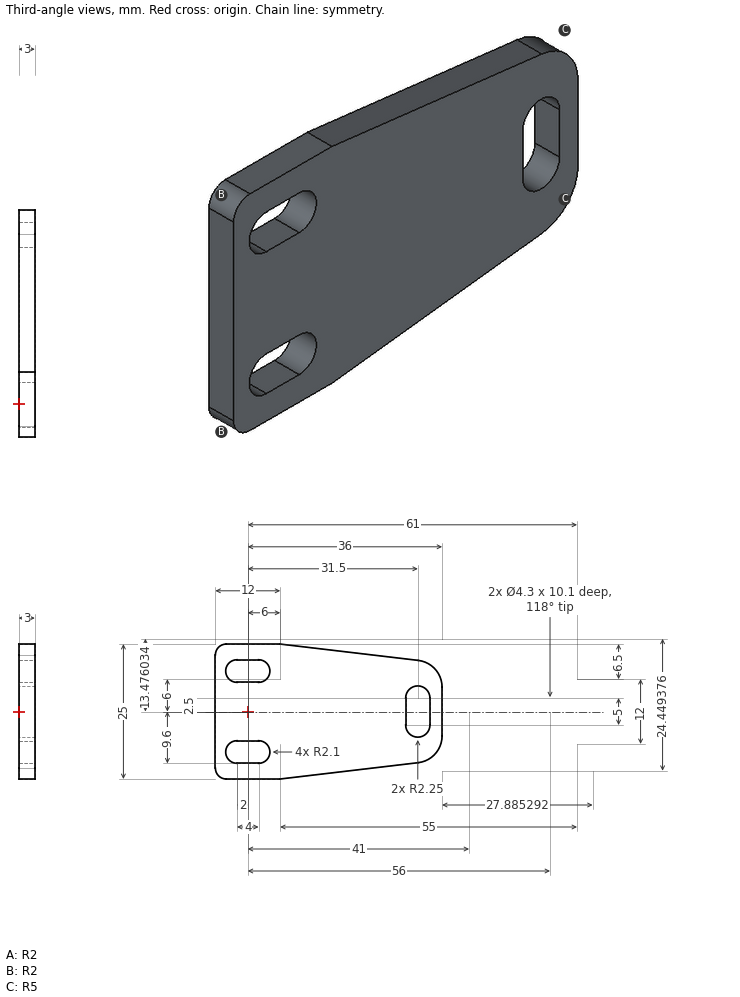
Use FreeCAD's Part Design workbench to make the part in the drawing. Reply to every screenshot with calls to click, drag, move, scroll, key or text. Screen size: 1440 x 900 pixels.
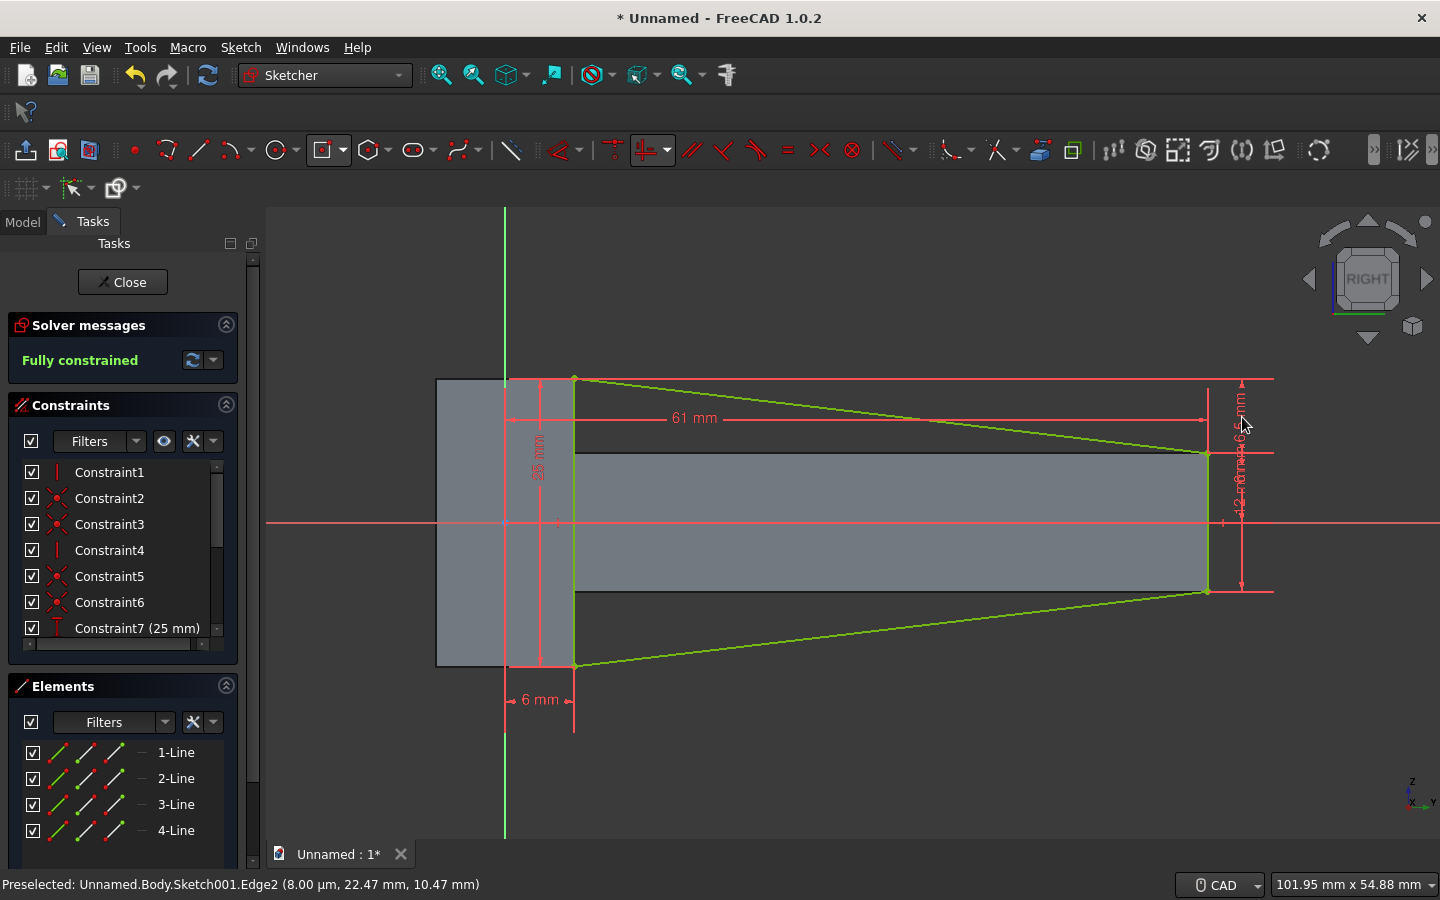
click(123, 282)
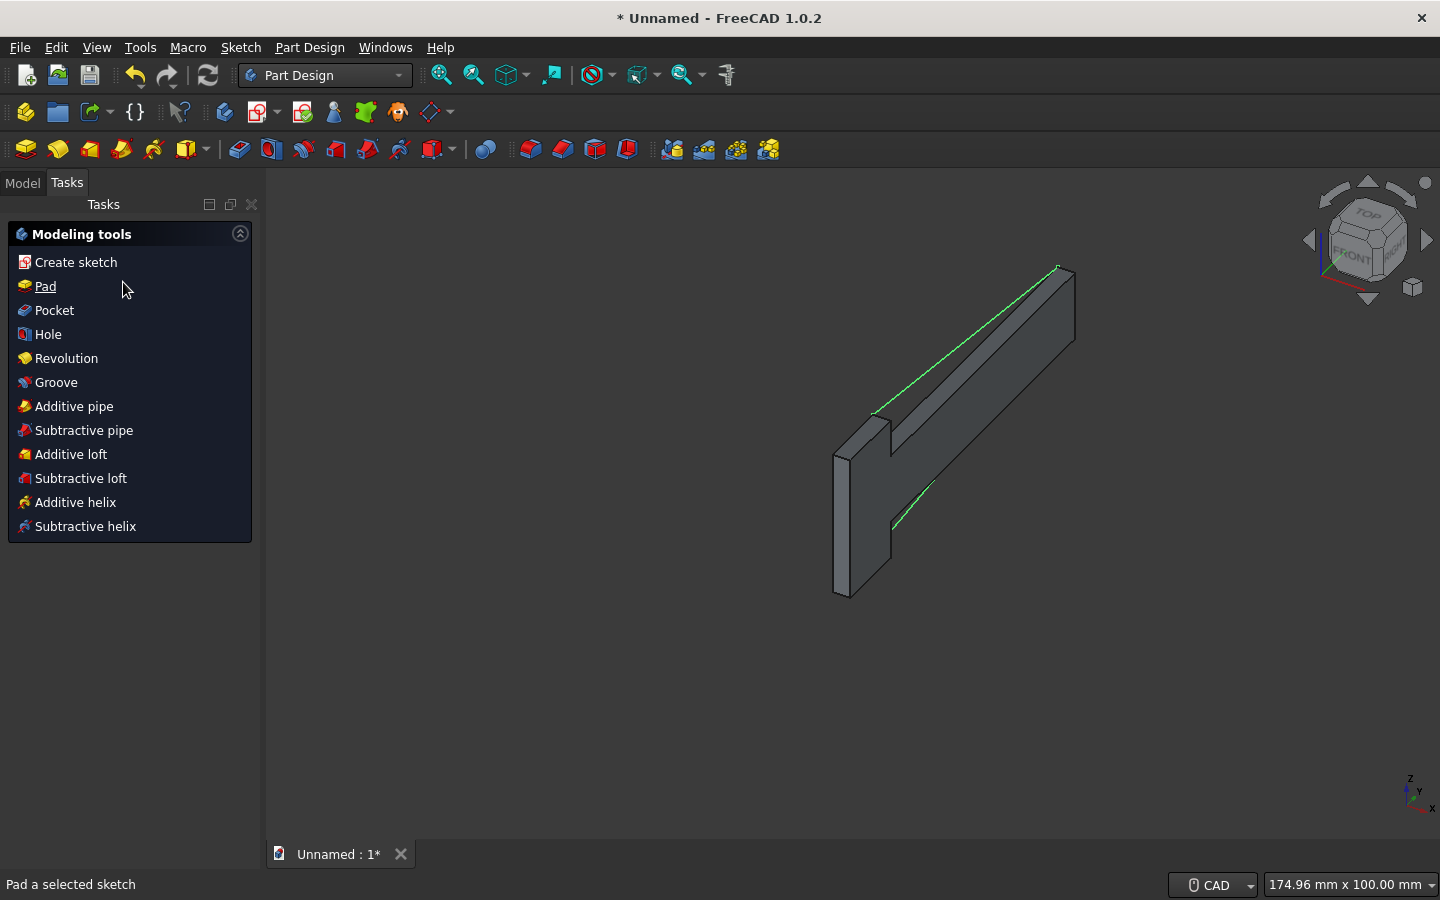
click(26, 150)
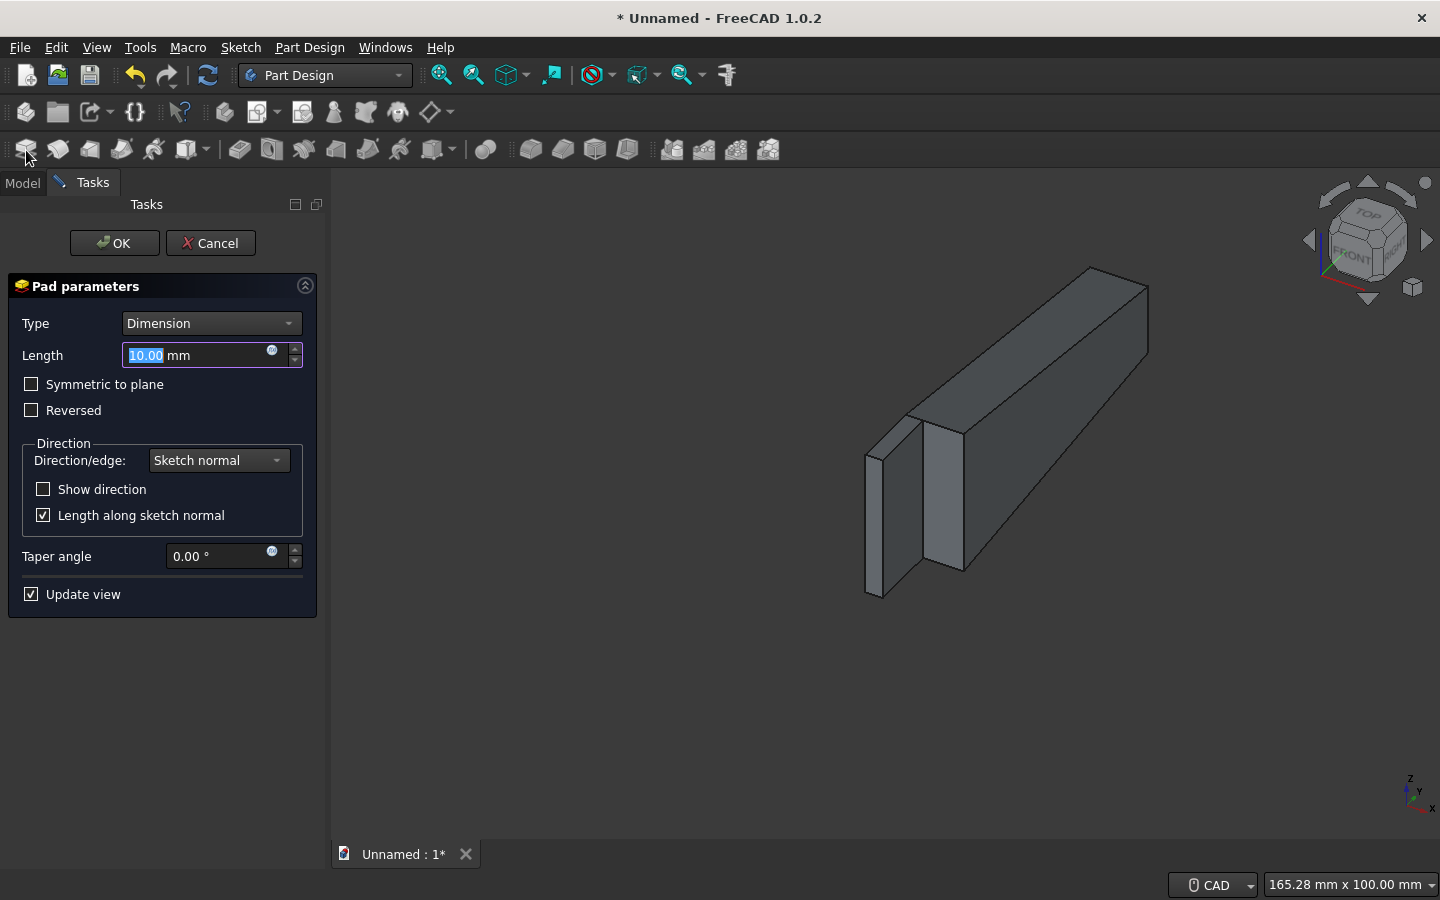
text(3)
key(Tab)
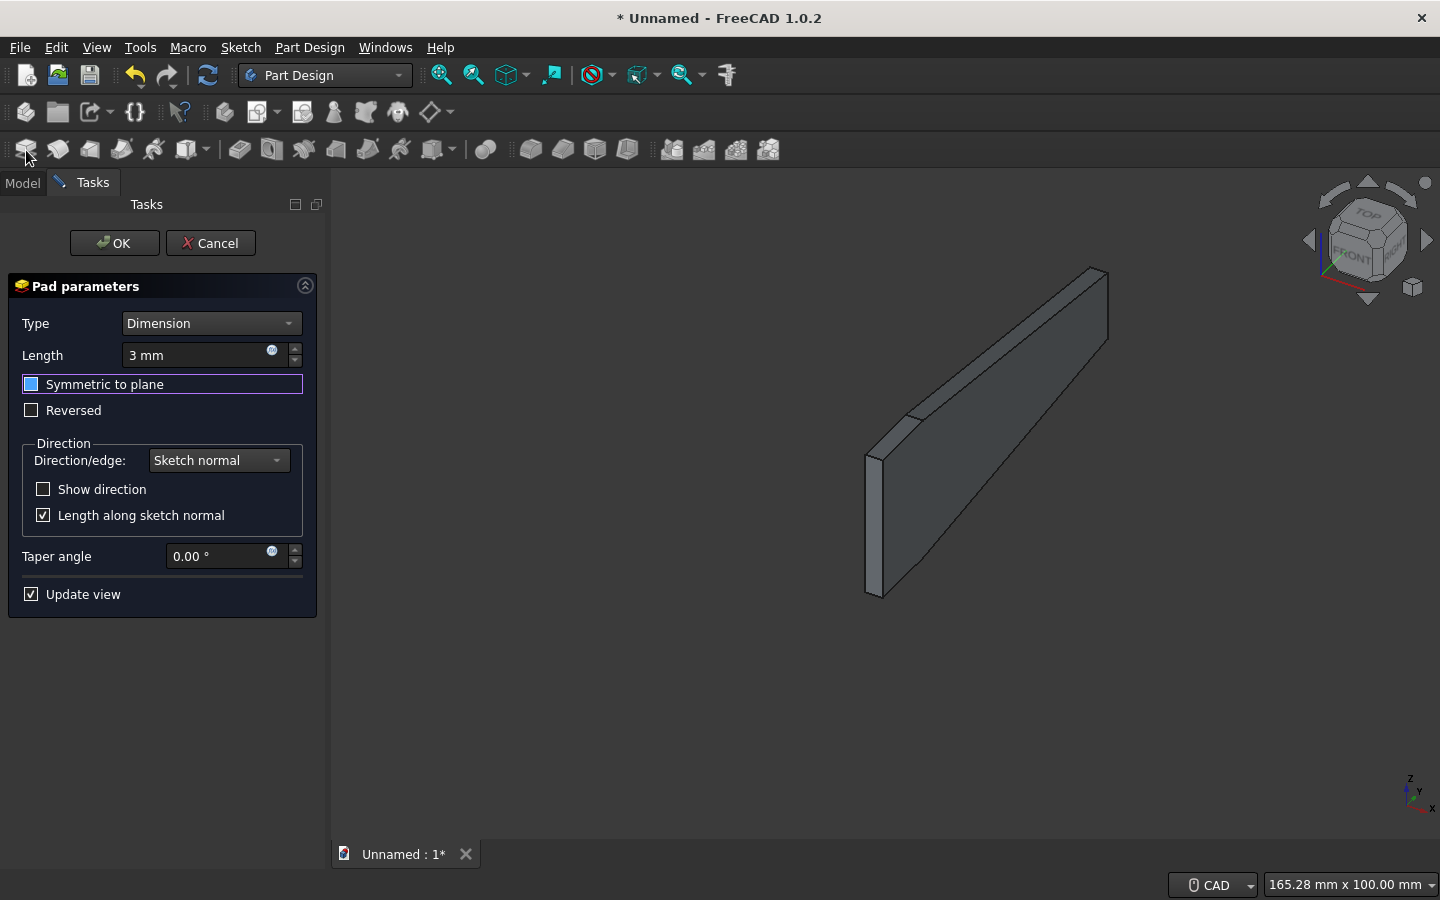
click(115, 243)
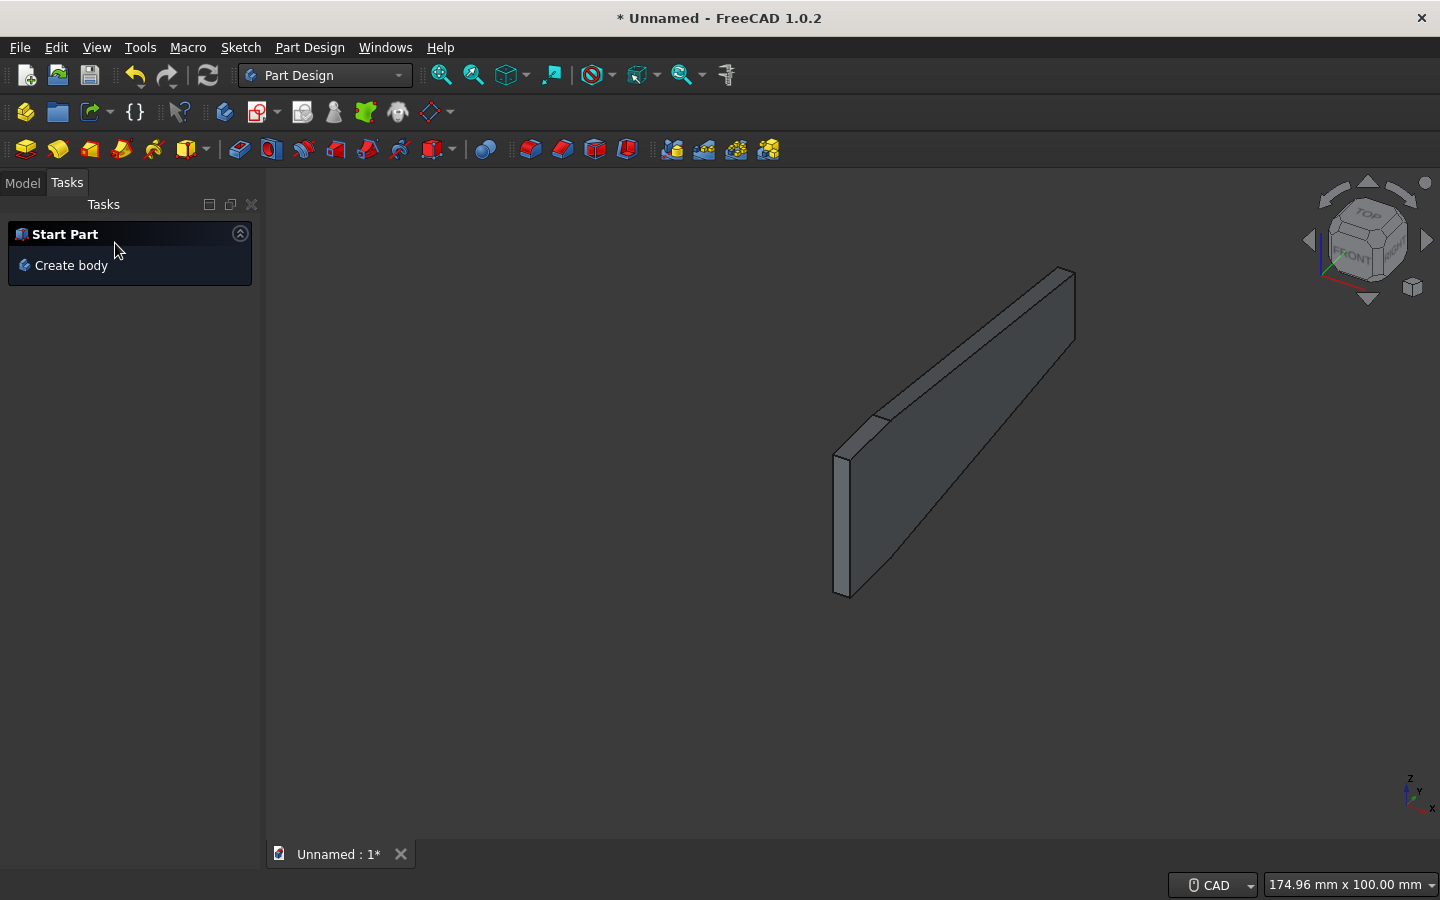
scroll(1066, 269, up, 4)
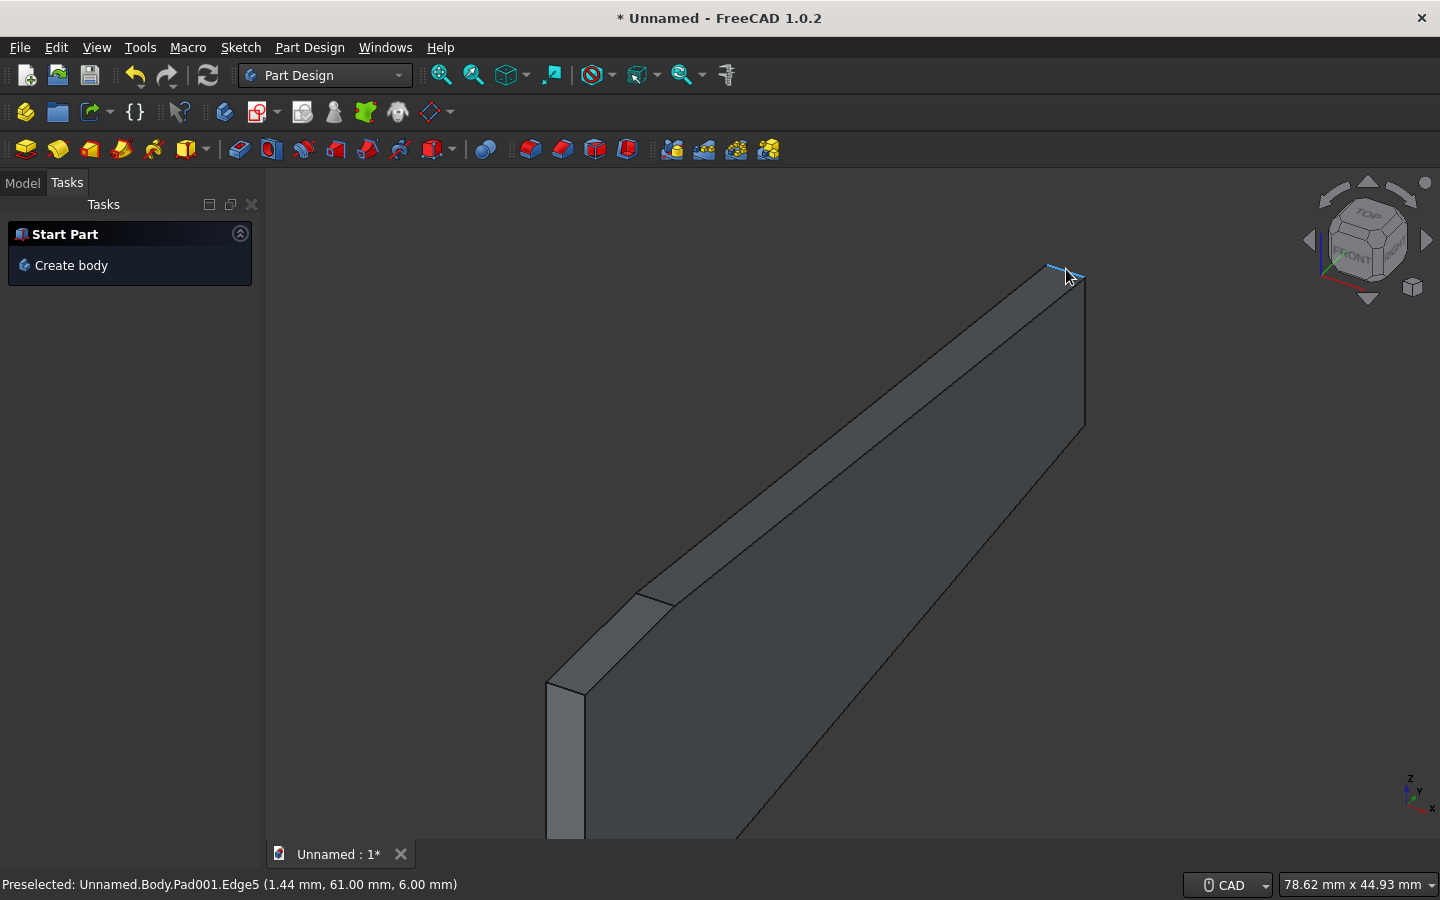
key(v)
key(f)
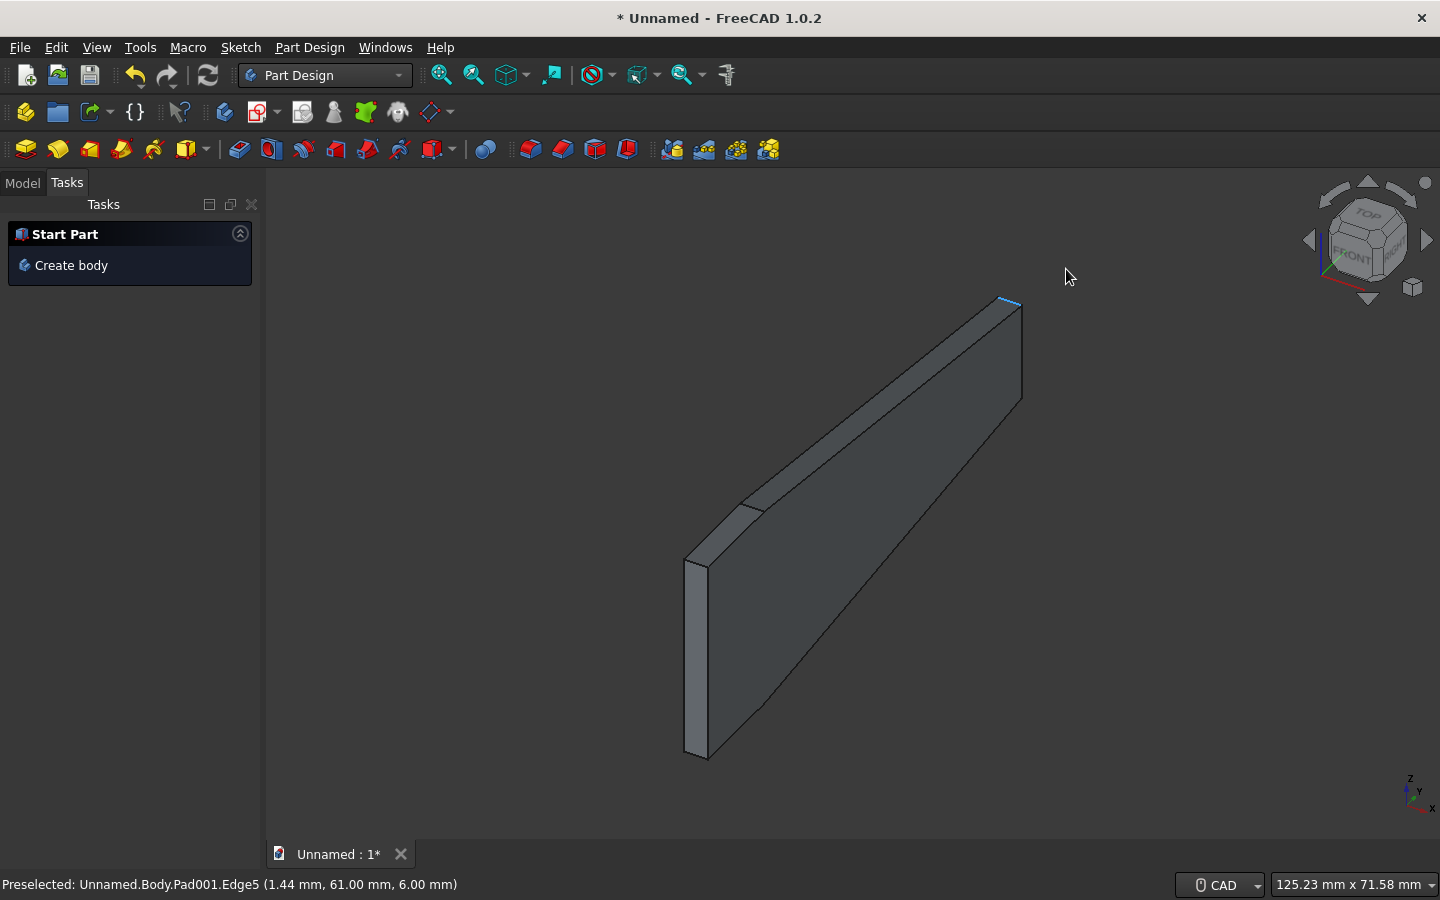
key(0)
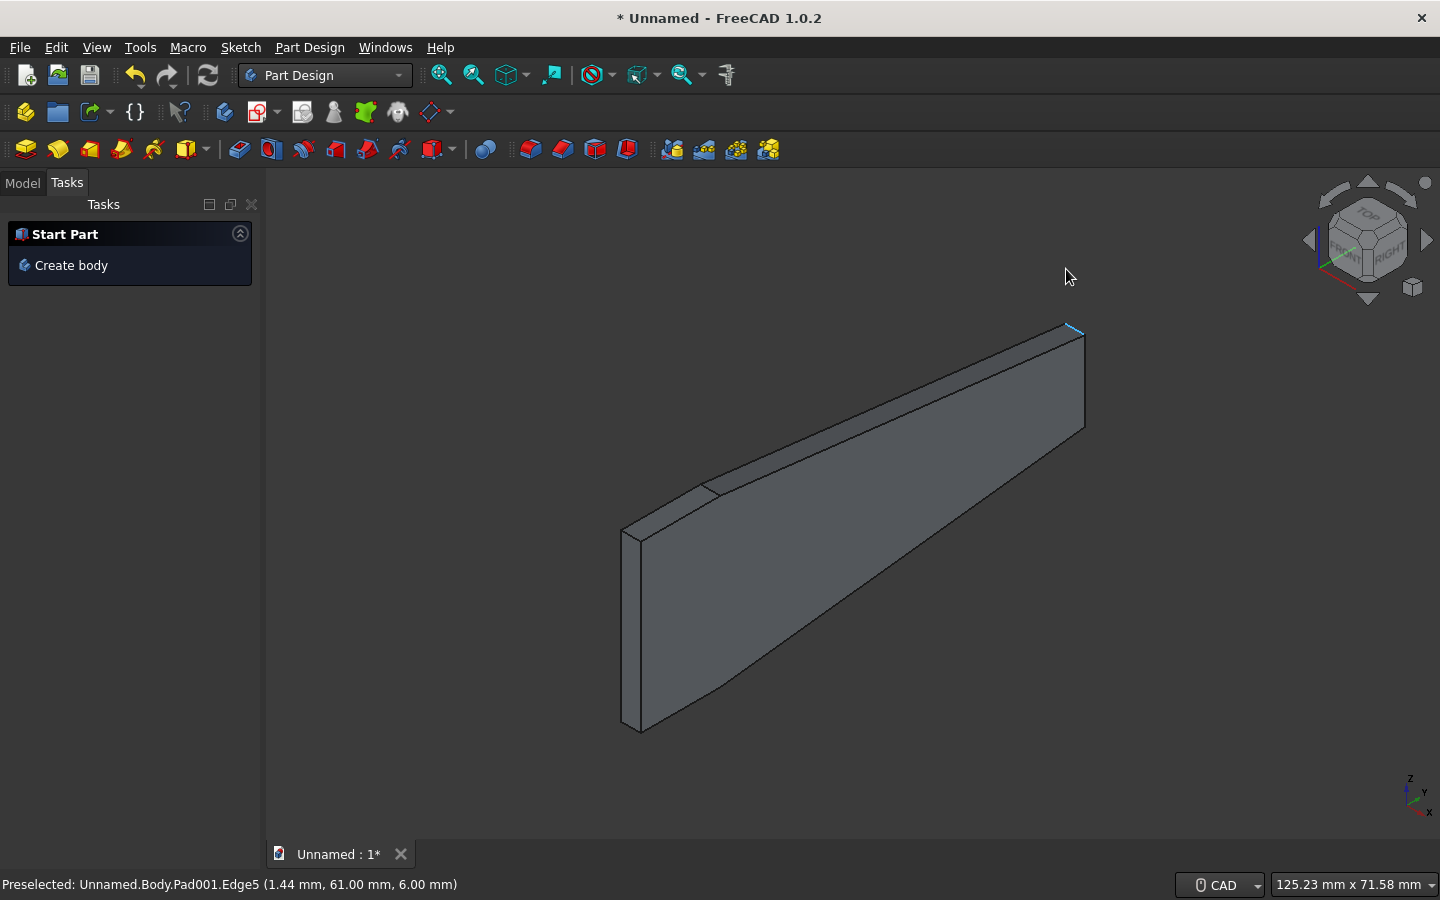
key(2)